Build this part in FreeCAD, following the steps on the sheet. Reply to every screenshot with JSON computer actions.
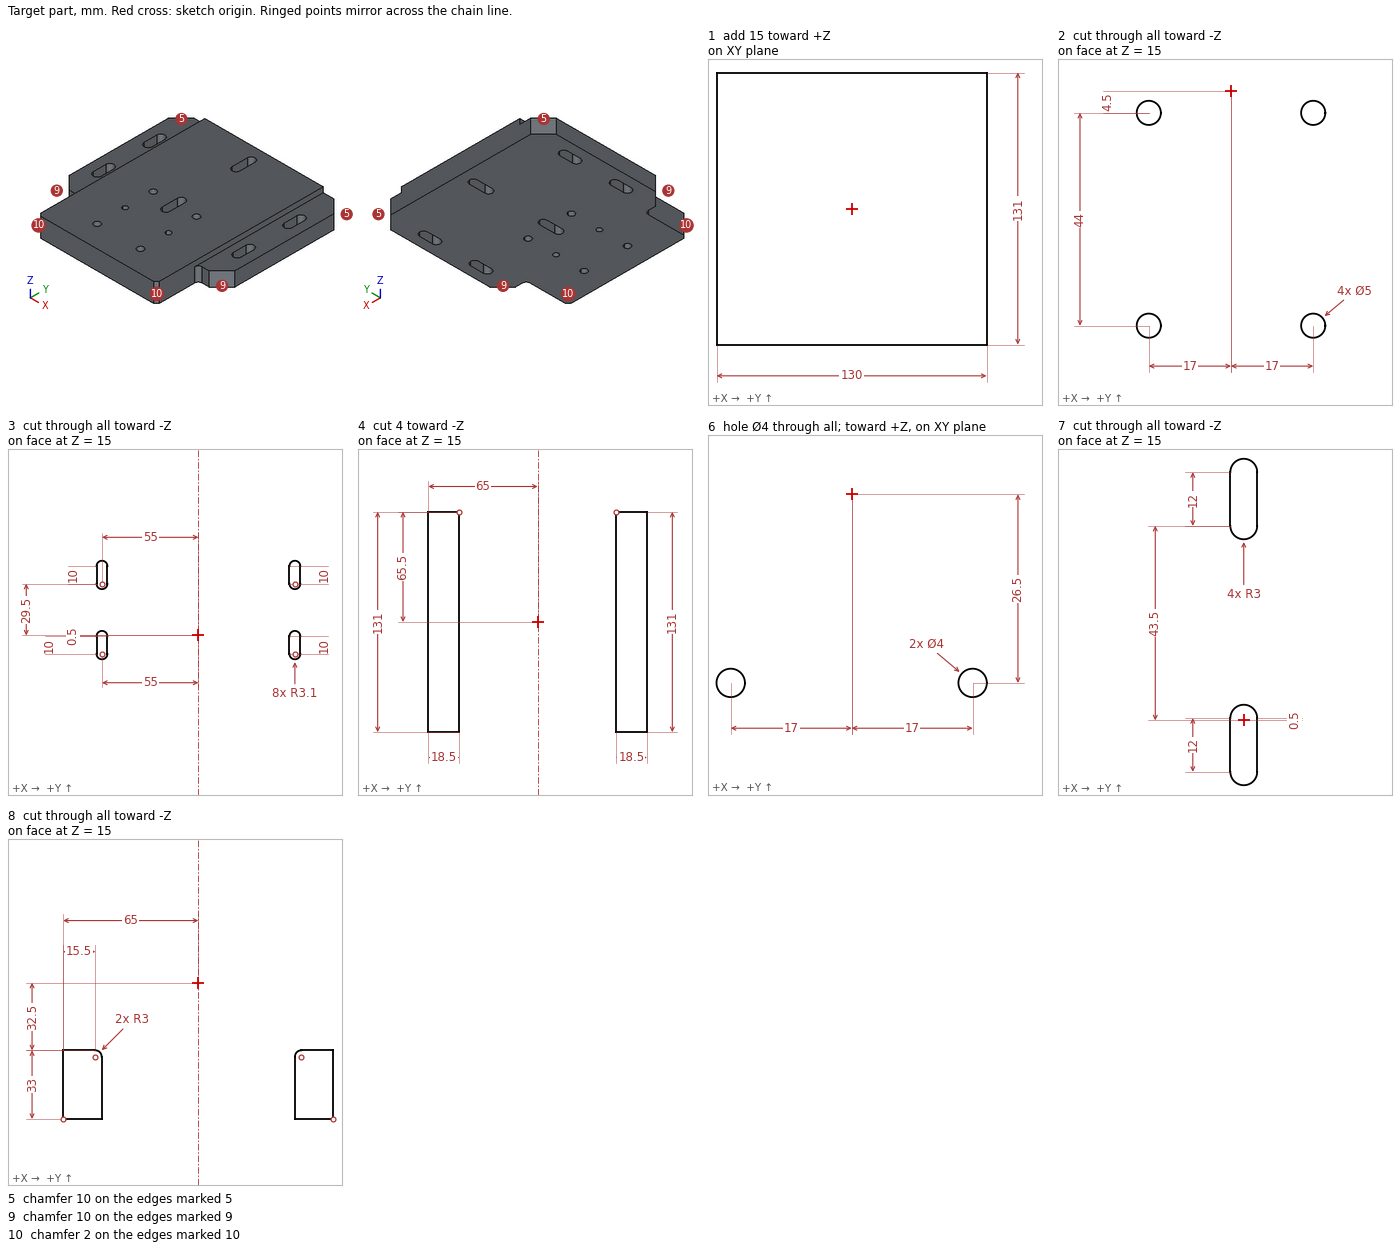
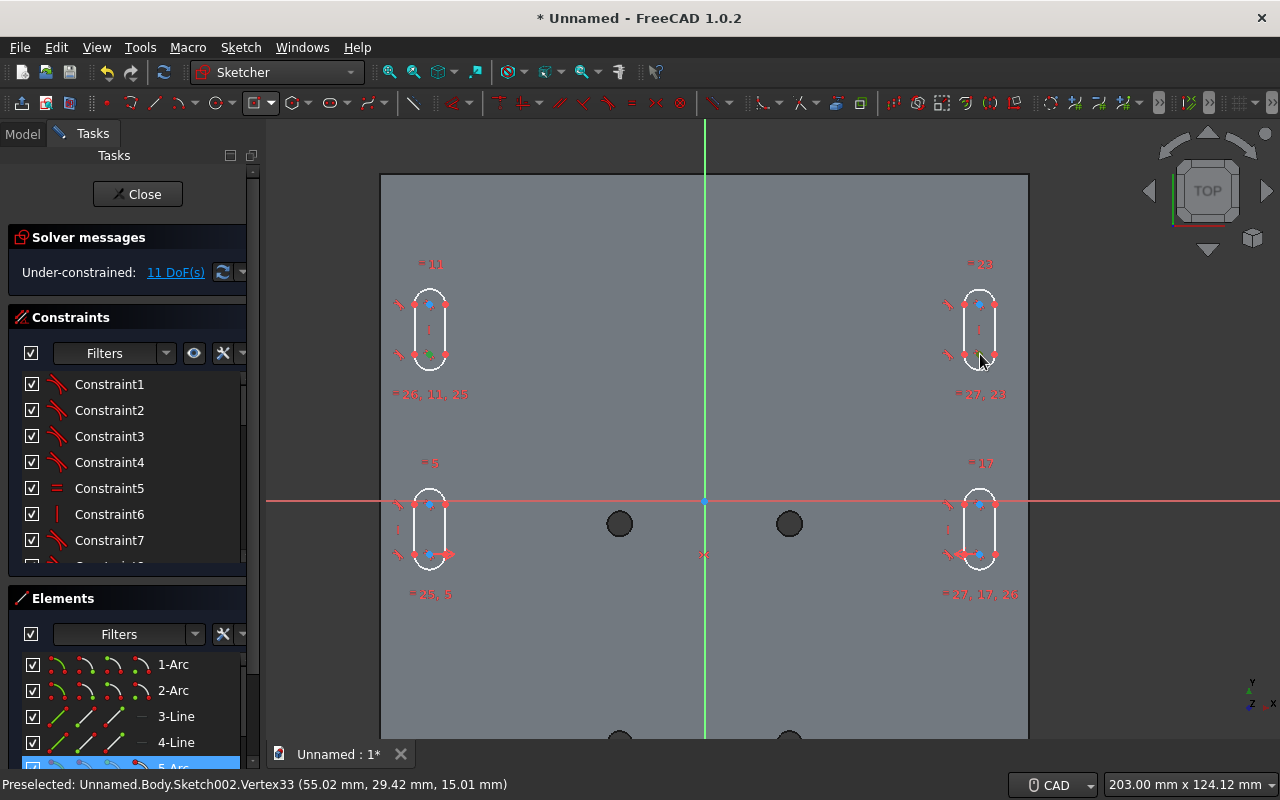
{"action": "left_click", "coordinate": [705, 671]}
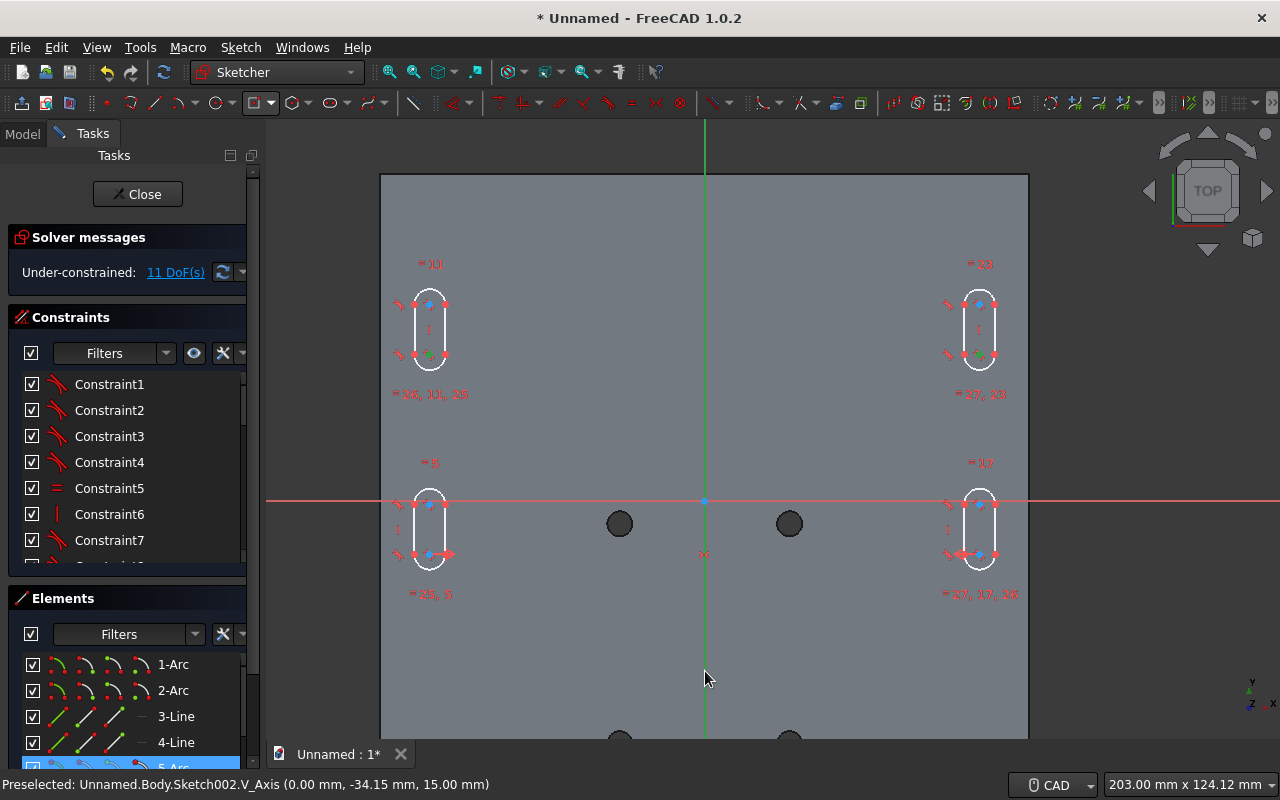
{"action": "key", "text": "s"}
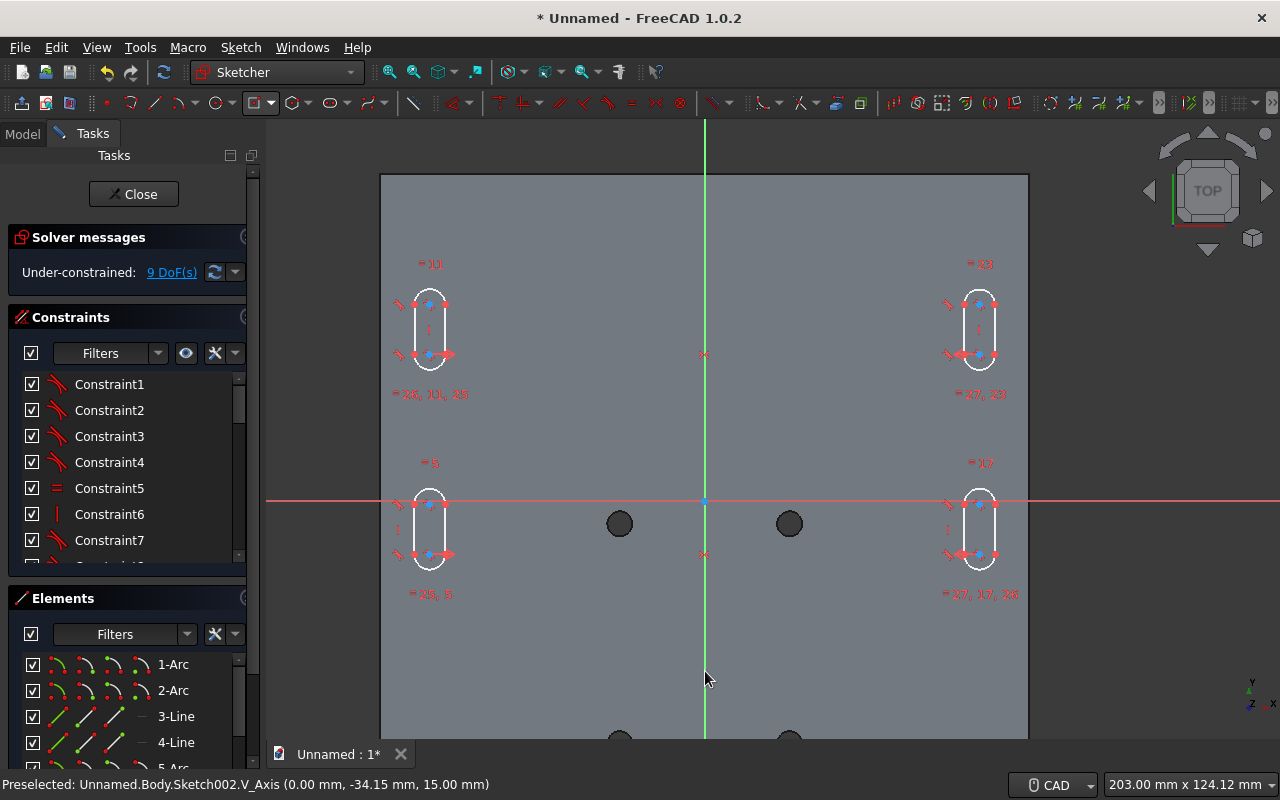
{"action": "left_click", "coordinate": [452, 104]}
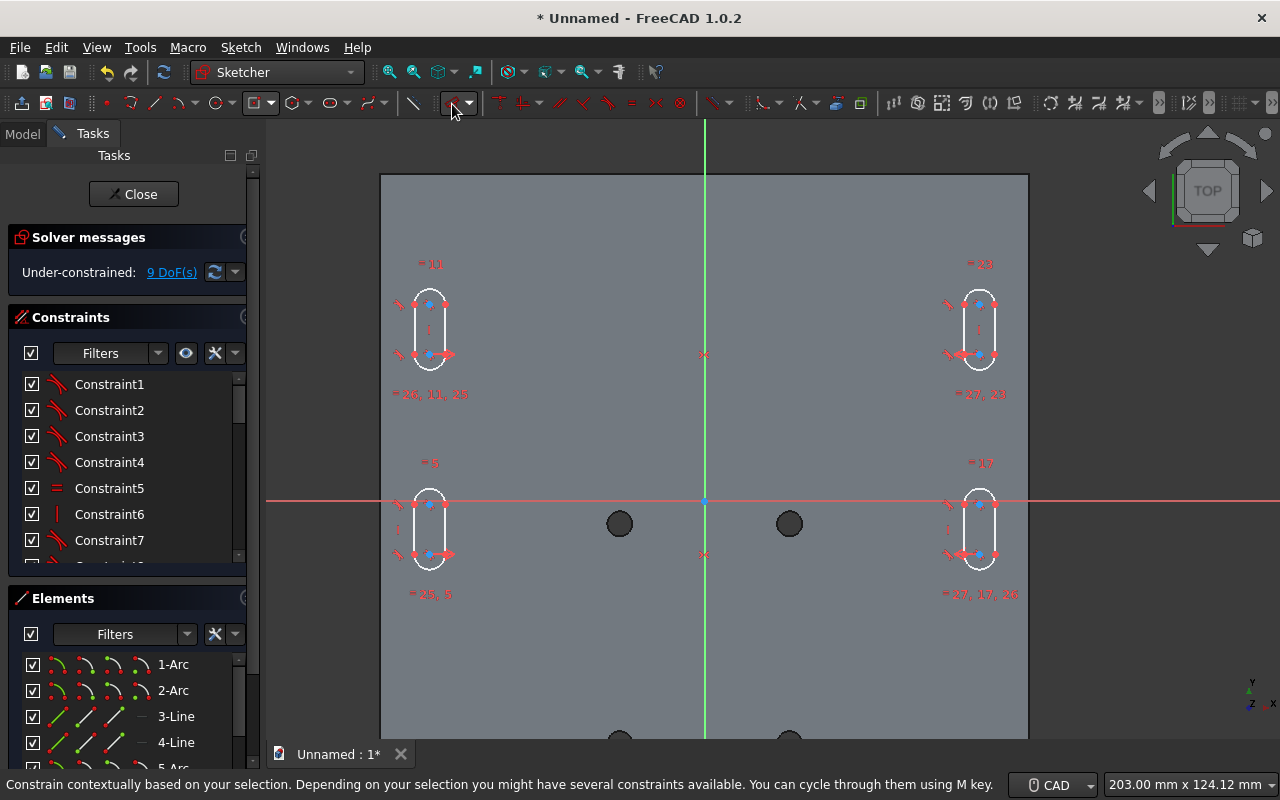
{"action": "scroll", "coordinate": [421, 567], "scroll_direction": "up", "scroll_amount": 5}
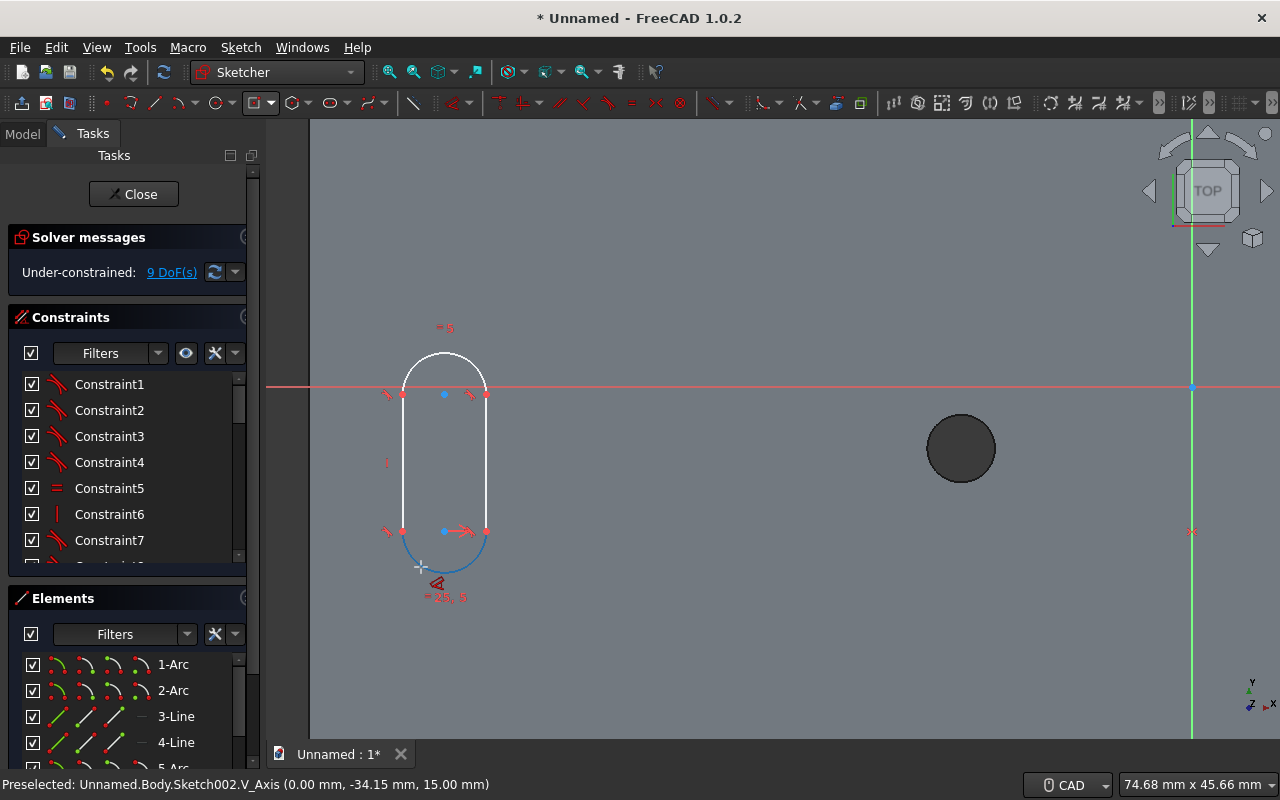
{"action": "left_click", "coordinate": [420, 565]}
{"action": "left_click", "coordinate": [401, 591]}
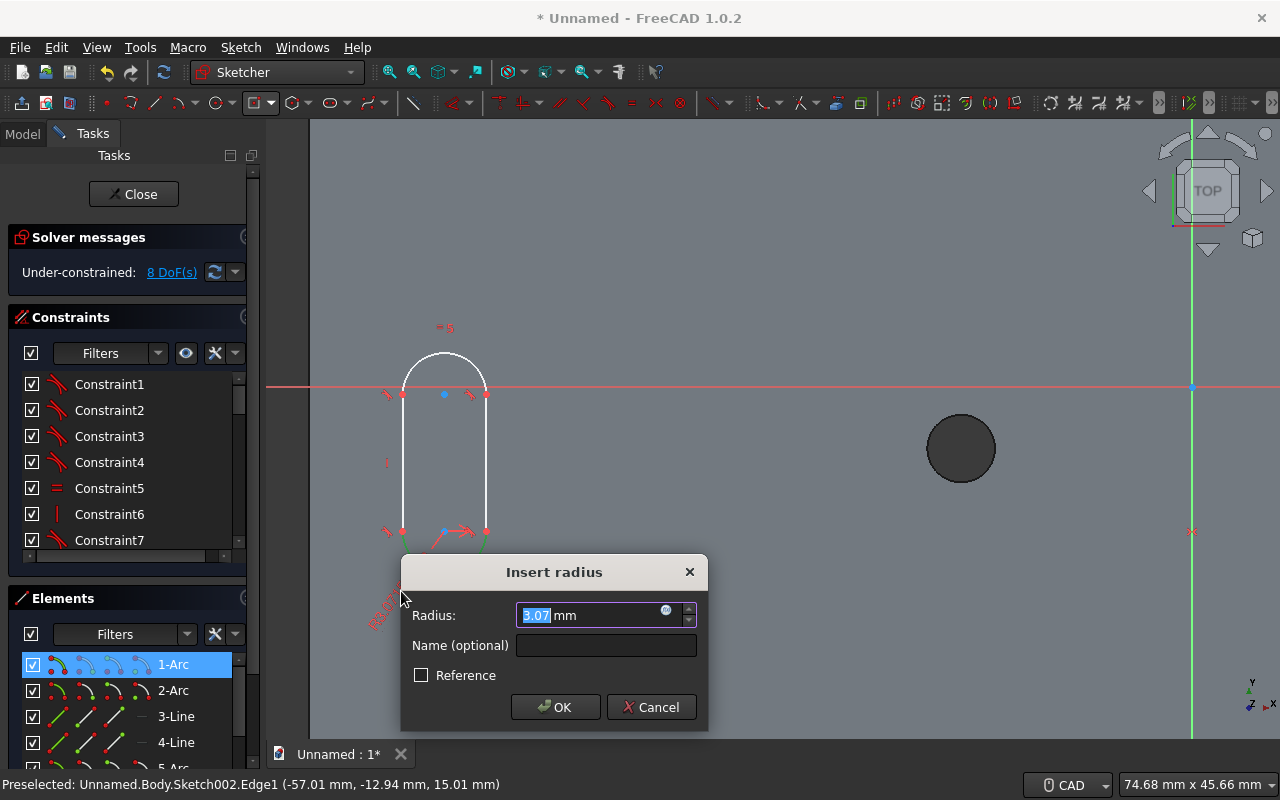
{"action": "type", "text": "3.1"}
{"action": "key", "text": "Return"}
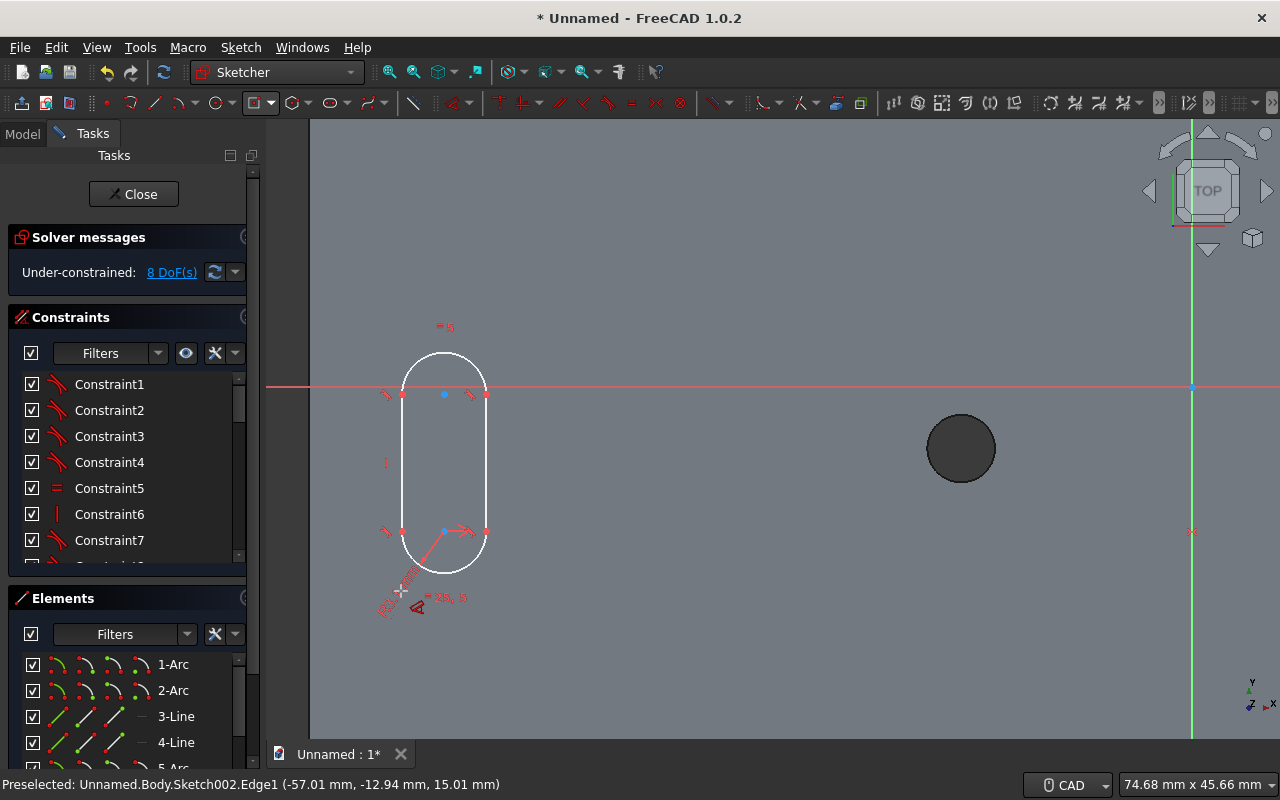
{"action": "left_click", "coordinate": [402, 490]}
{"action": "left_click", "coordinate": [368, 463]}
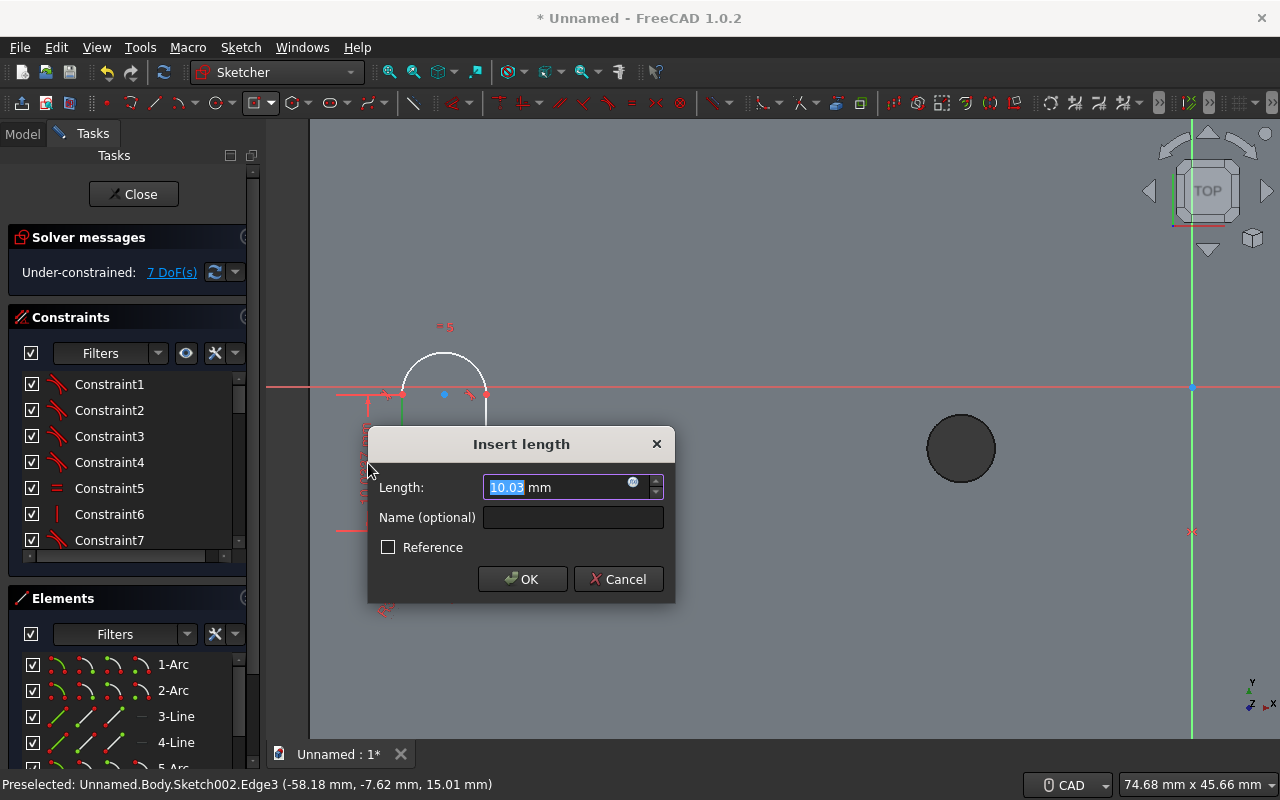
{"action": "type", "text": "10"}
{"action": "key", "text": "Return"}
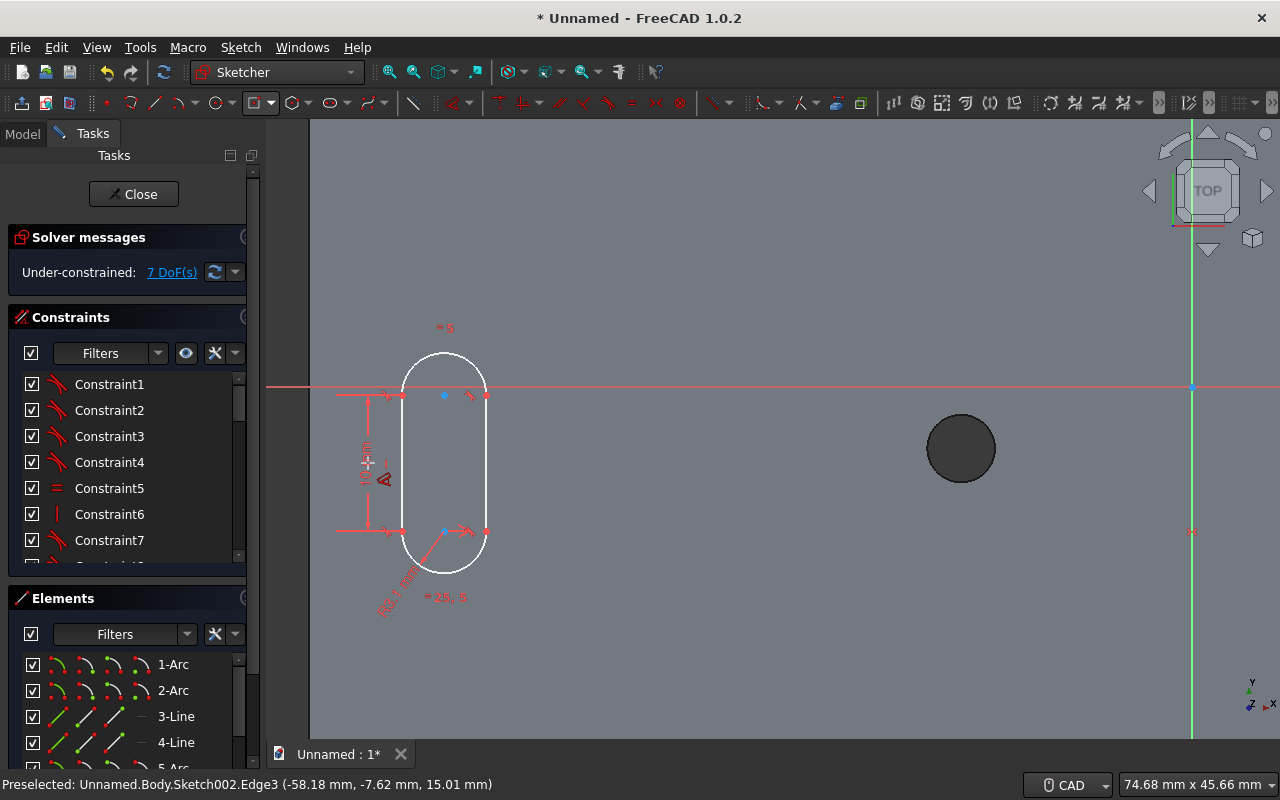
{"action": "scroll", "coordinate": [421, 568], "scroll_direction": "down", "scroll_amount": 5}